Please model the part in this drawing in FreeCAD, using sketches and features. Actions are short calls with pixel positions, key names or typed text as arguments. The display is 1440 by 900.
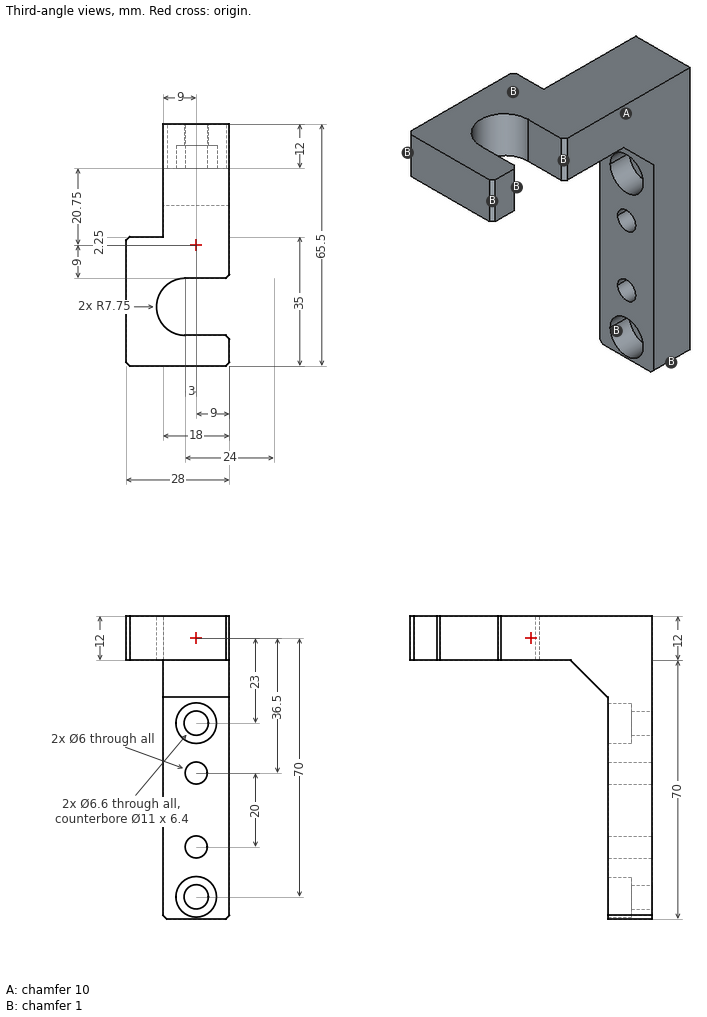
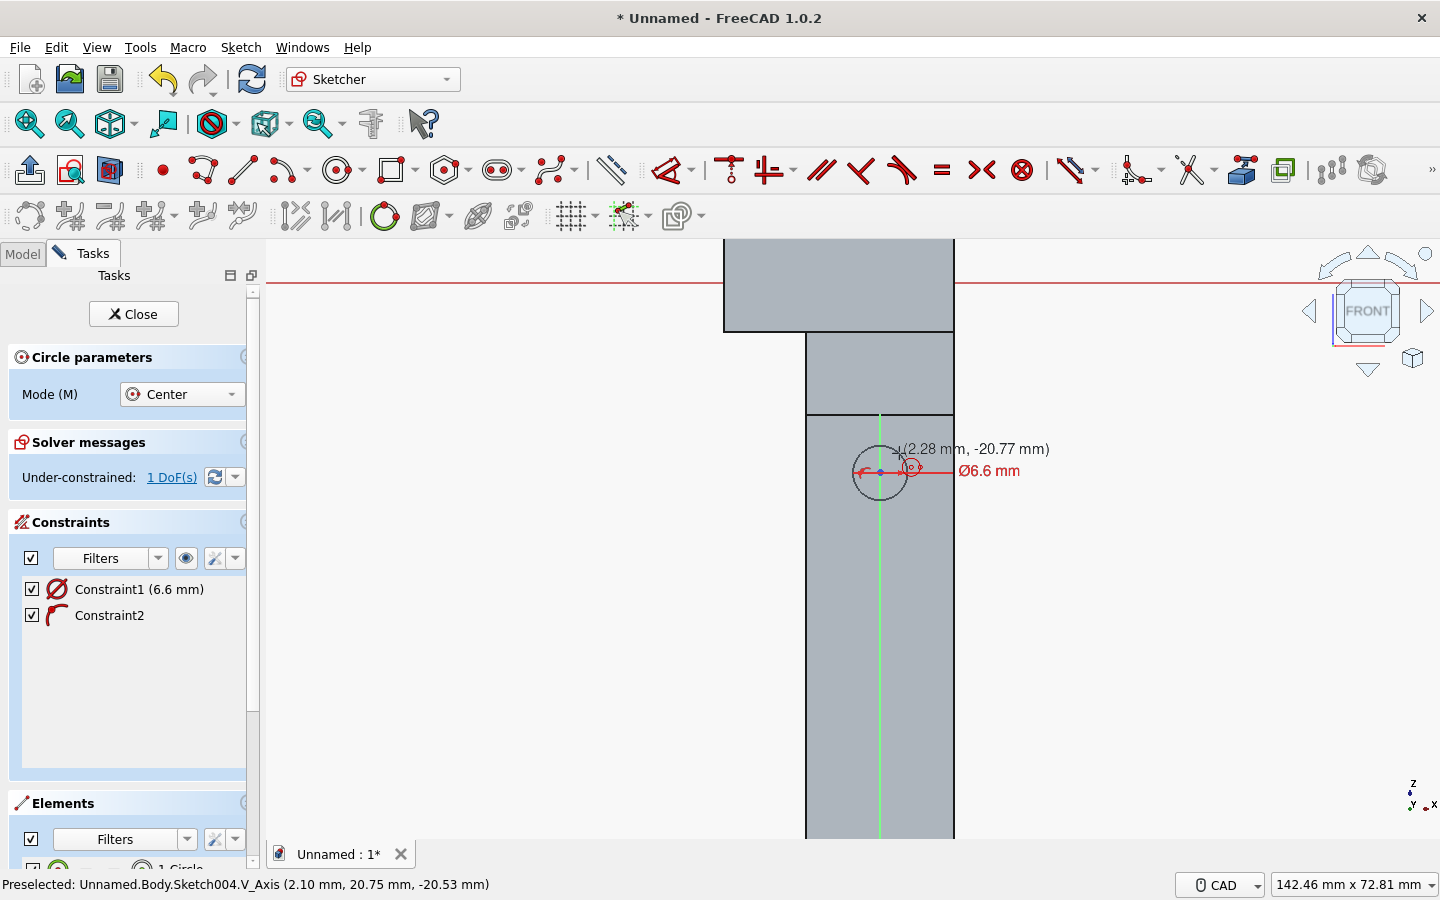
scroll(590, 446, down, 2)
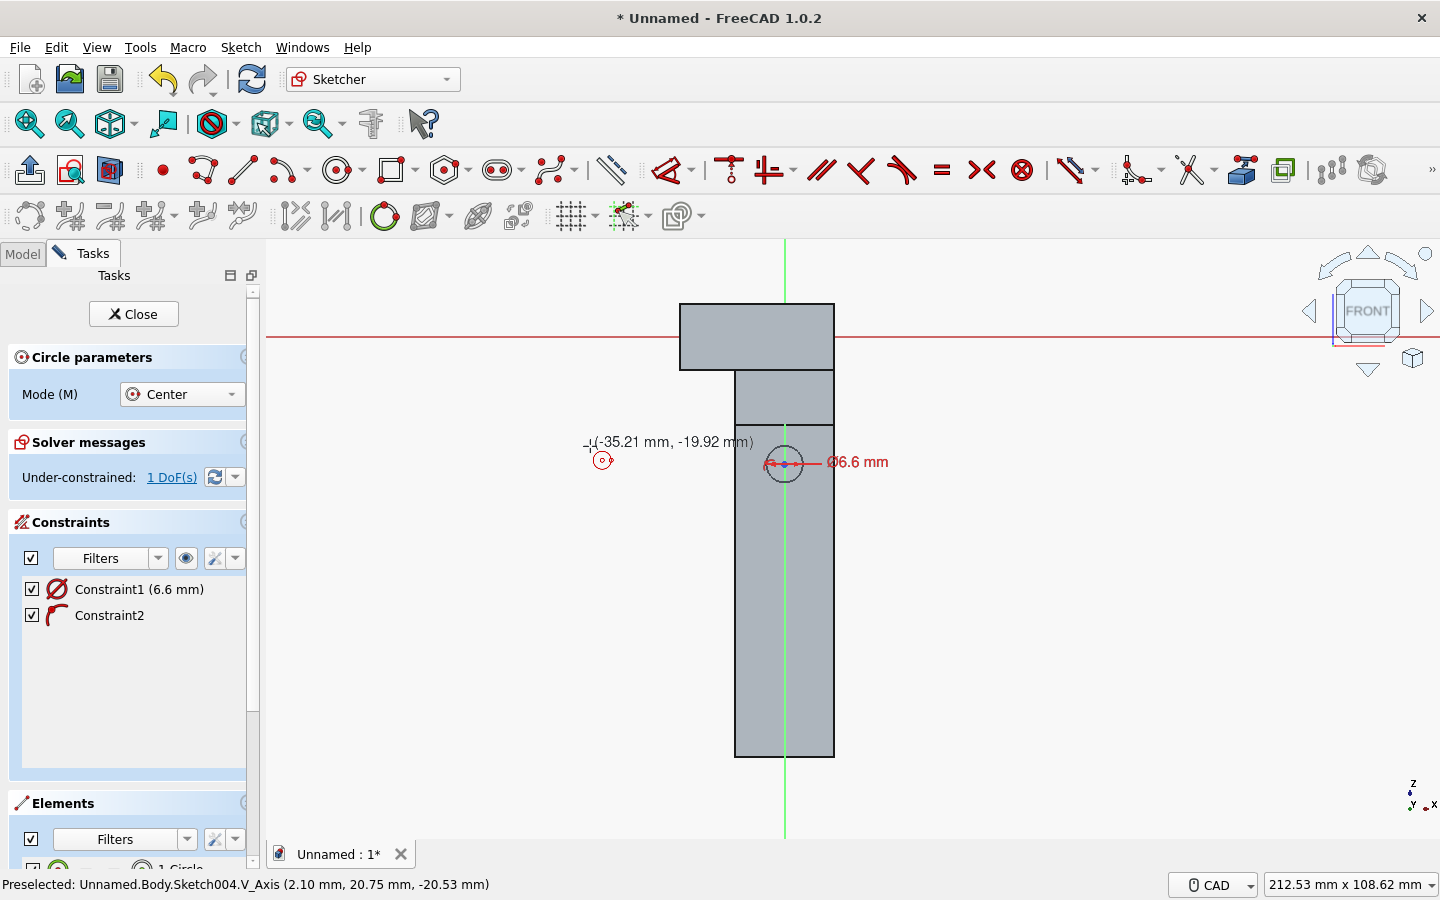
scroll(785, 723, up, 2)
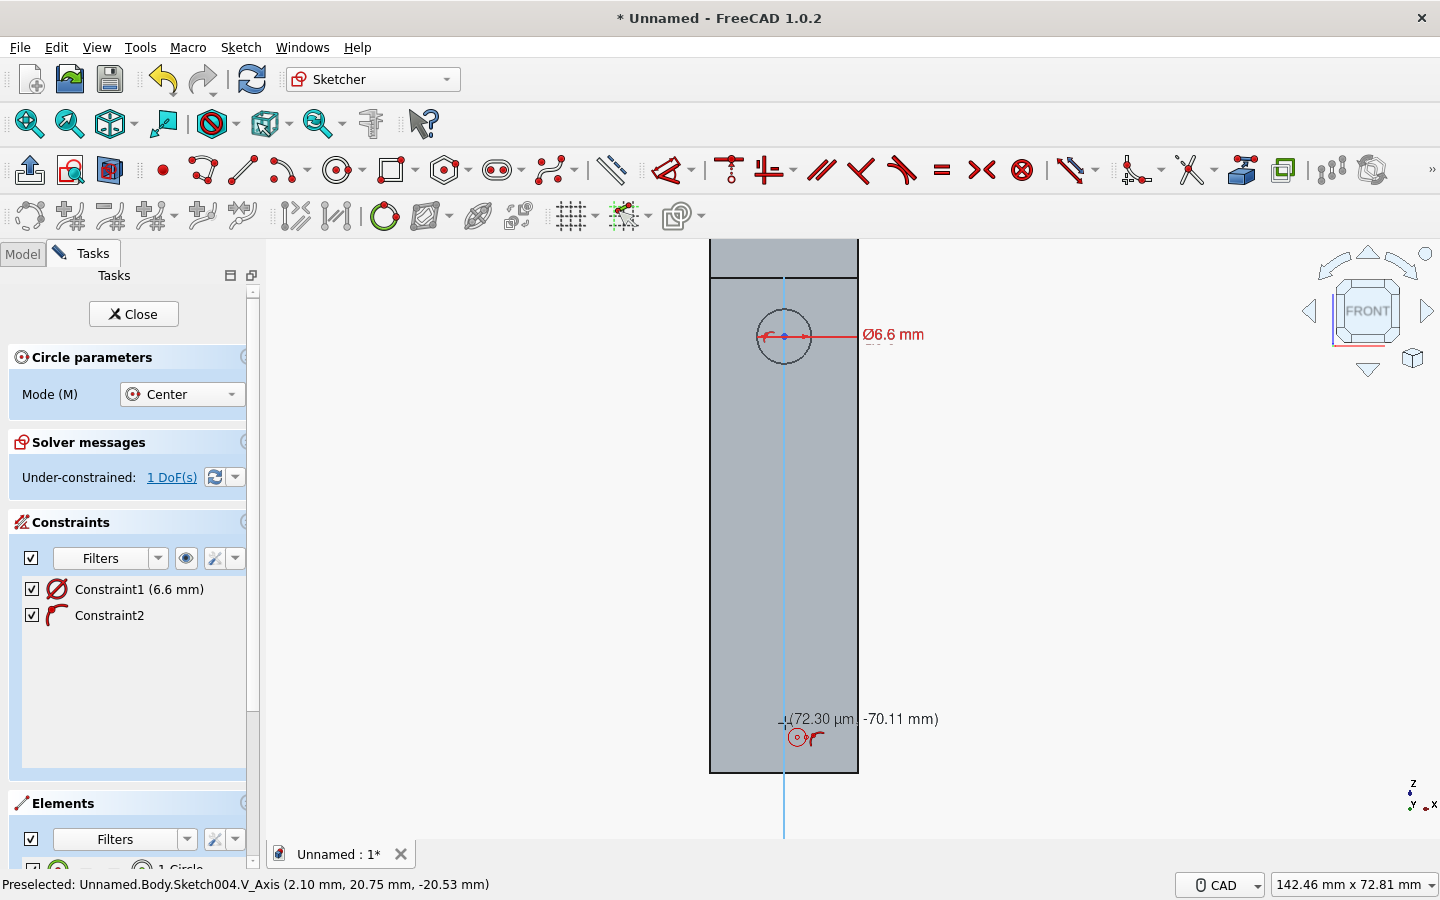
click(784, 723)
move(803, 704)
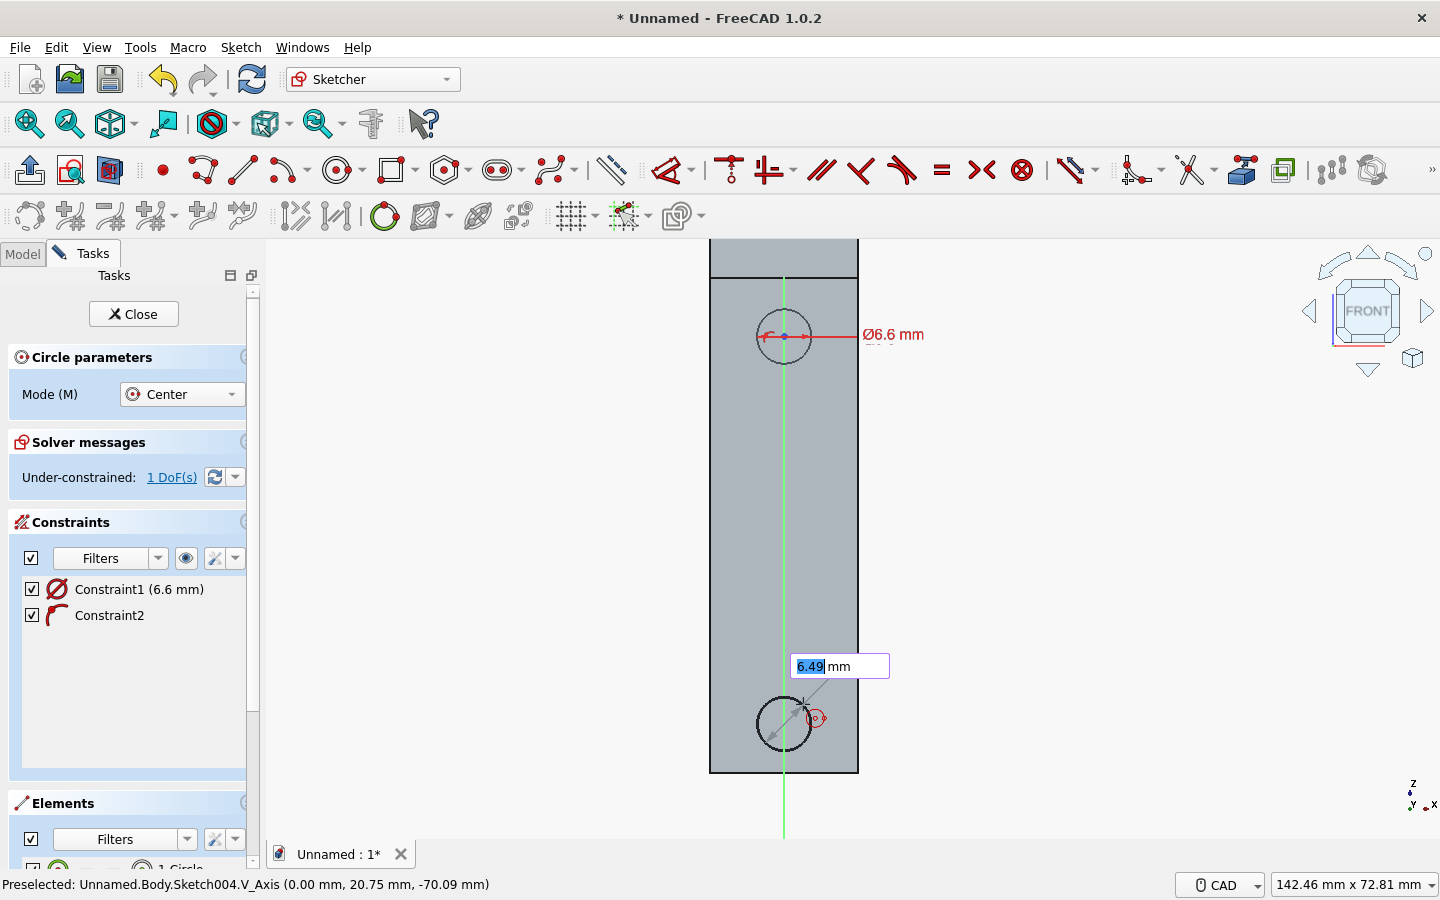
text(6.6)
key(Return)
key(Escape)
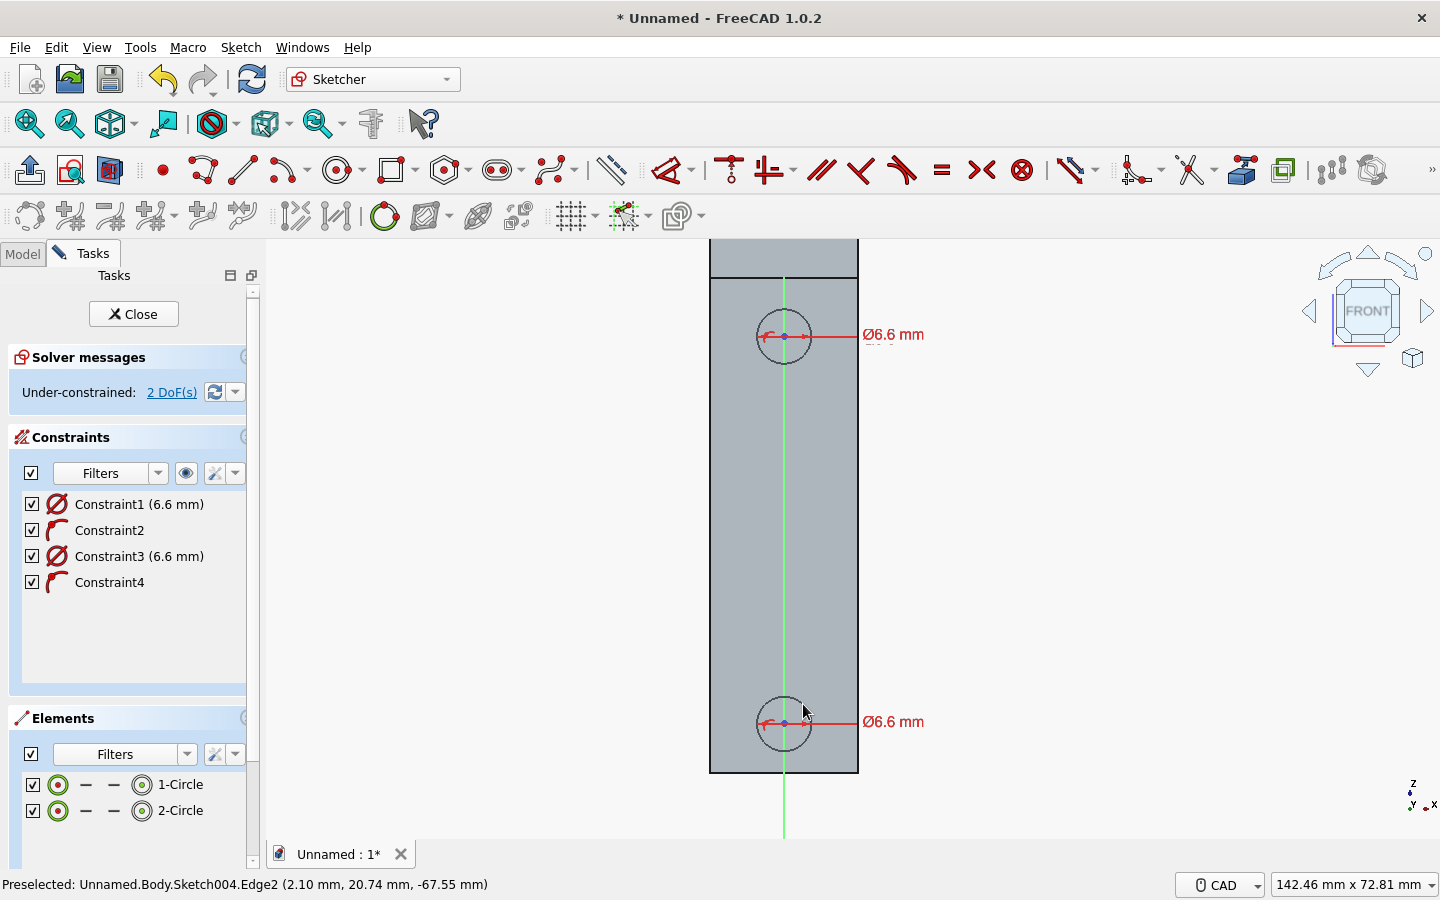
key(d)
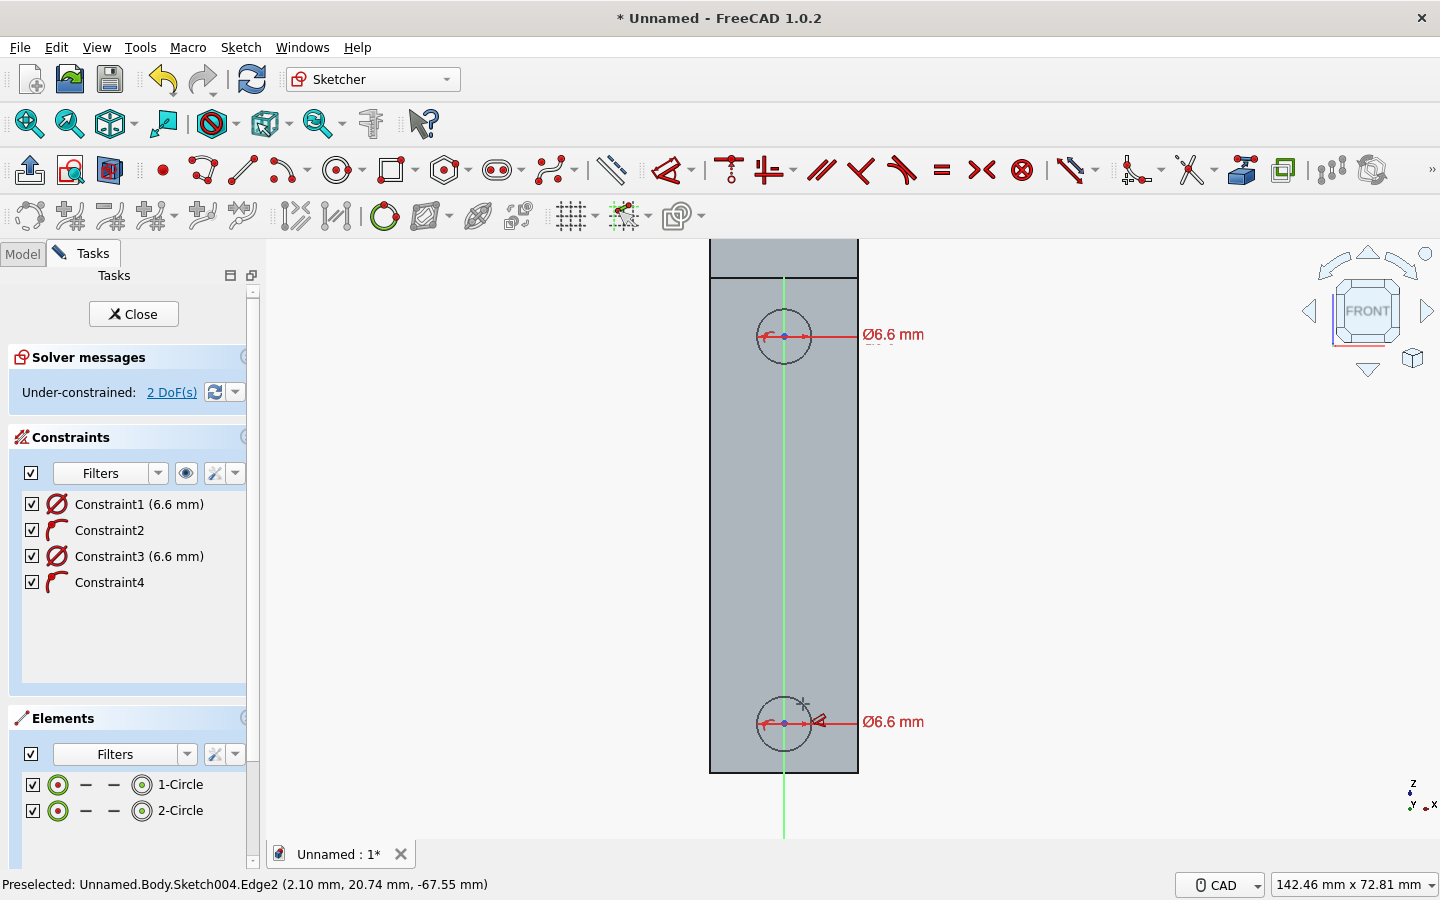
click(784, 337)
click(818, 302)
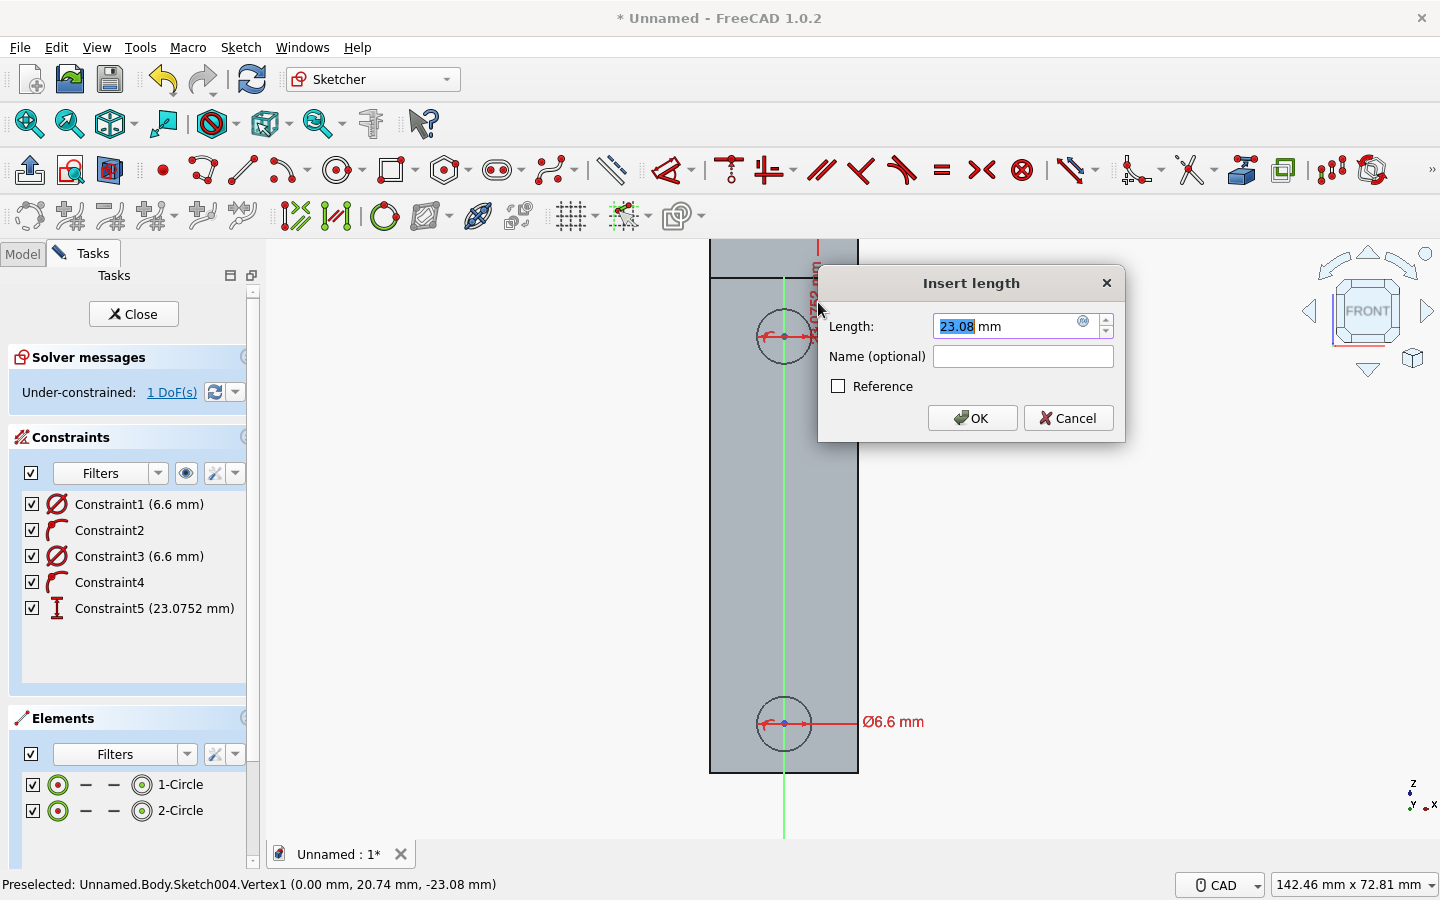
text(23)
key(Return)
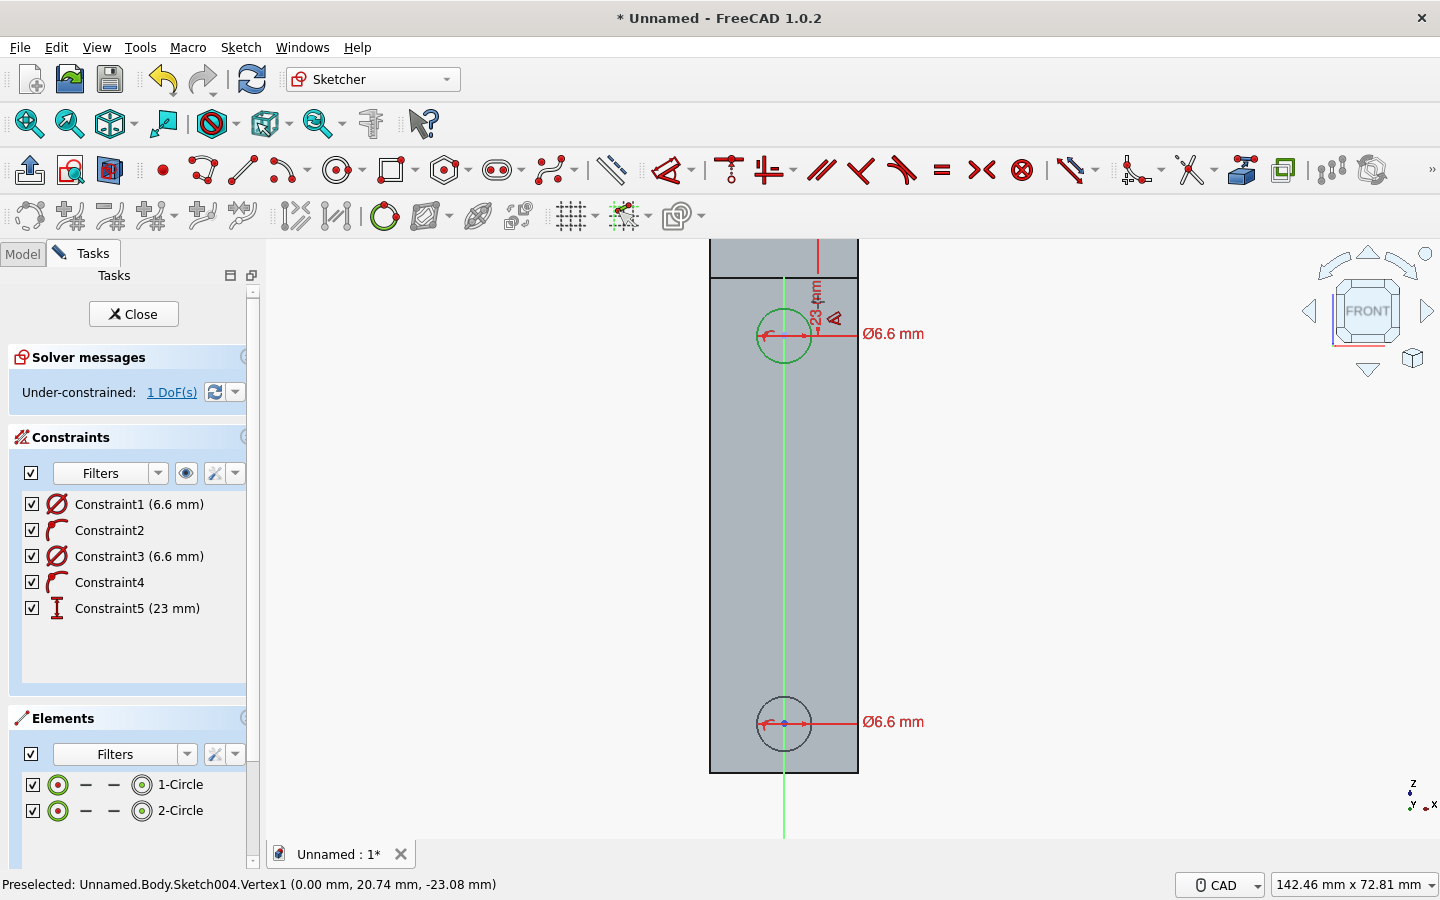
click(784, 724)
click(818, 496)